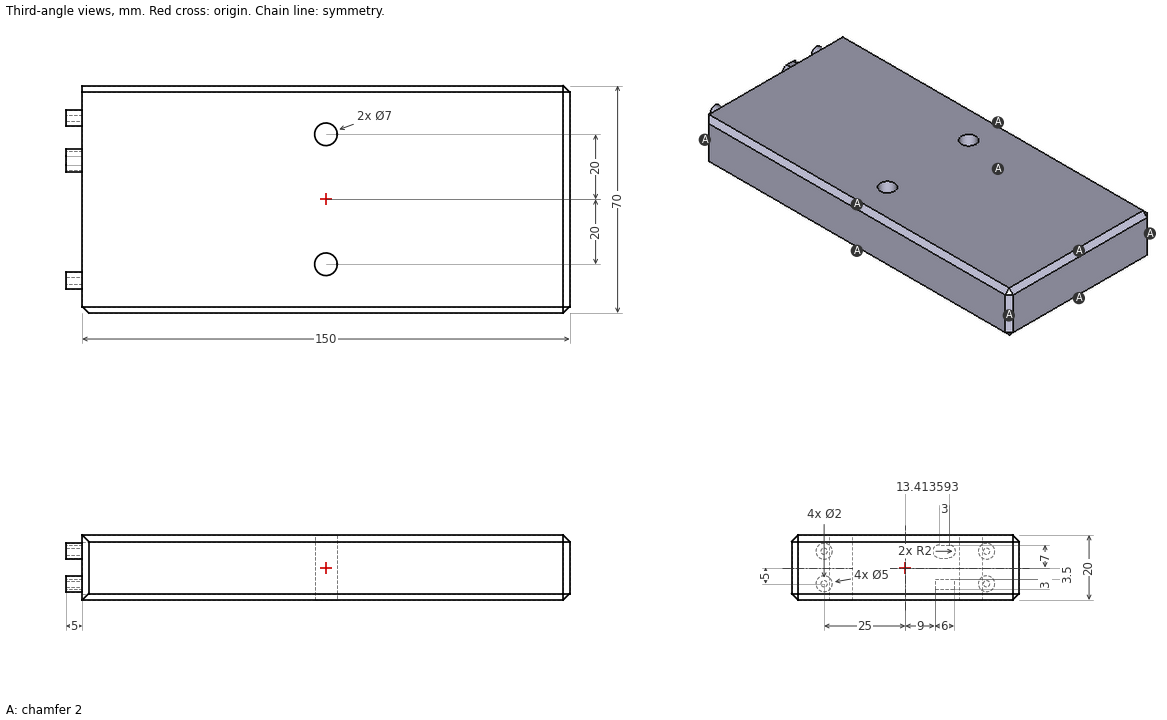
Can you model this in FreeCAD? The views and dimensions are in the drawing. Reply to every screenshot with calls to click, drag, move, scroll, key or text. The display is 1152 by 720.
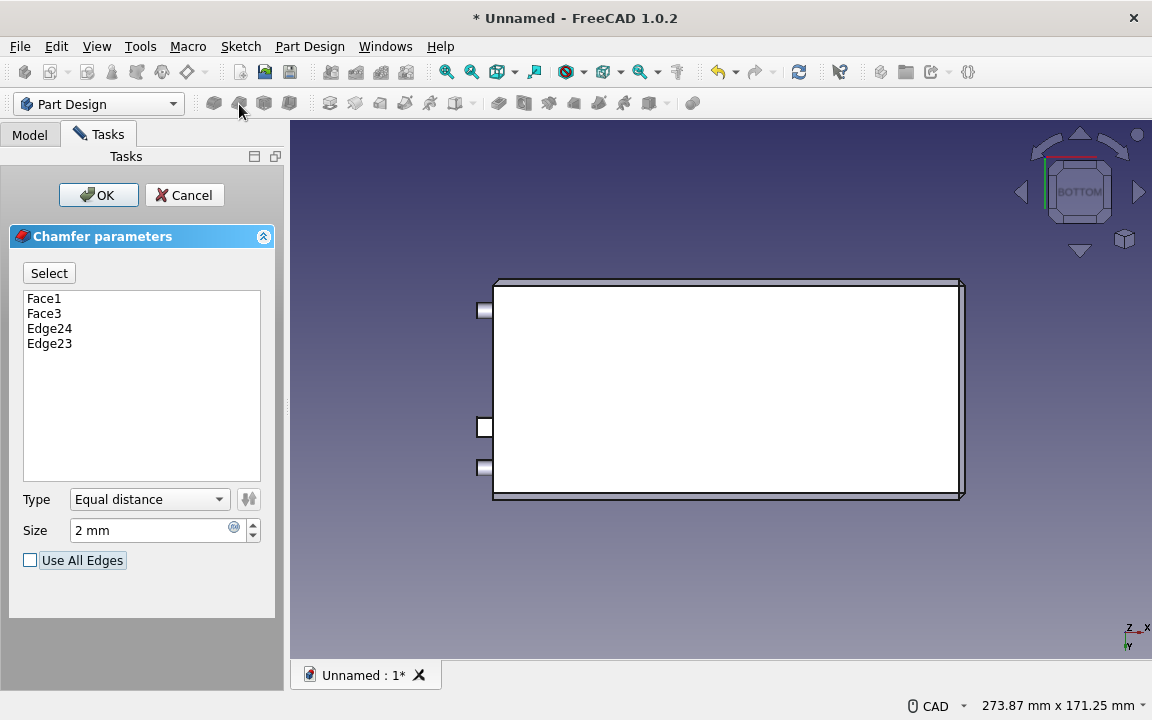
click(99, 195)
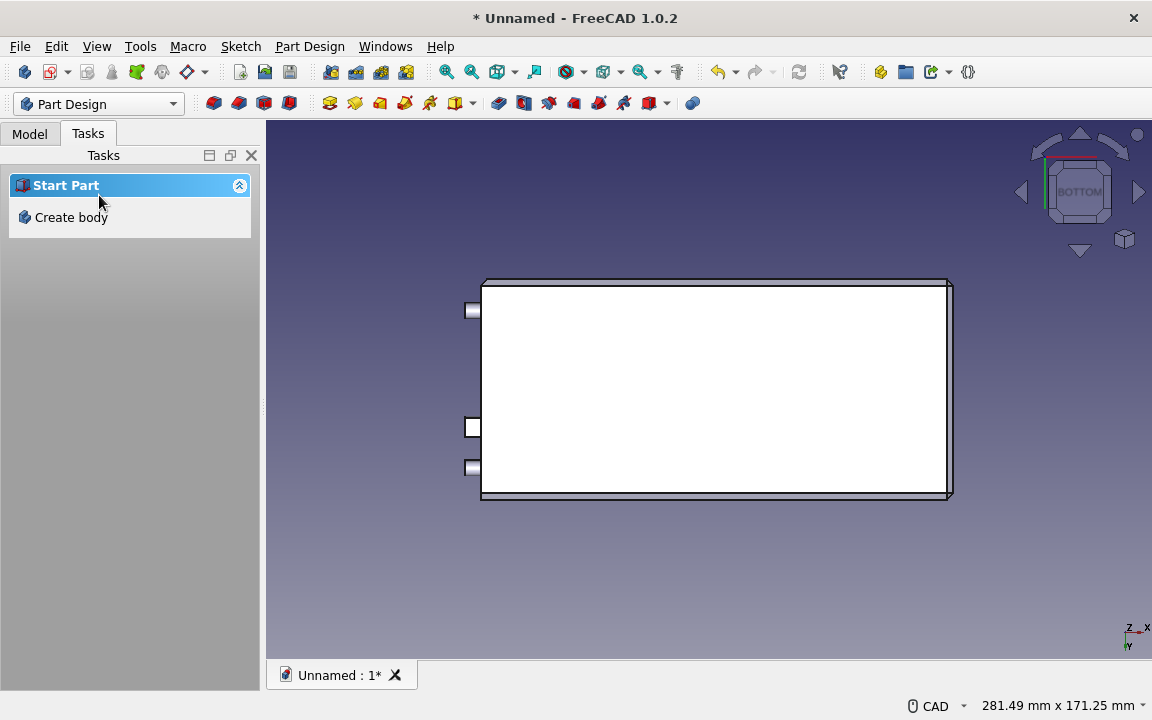
key(0)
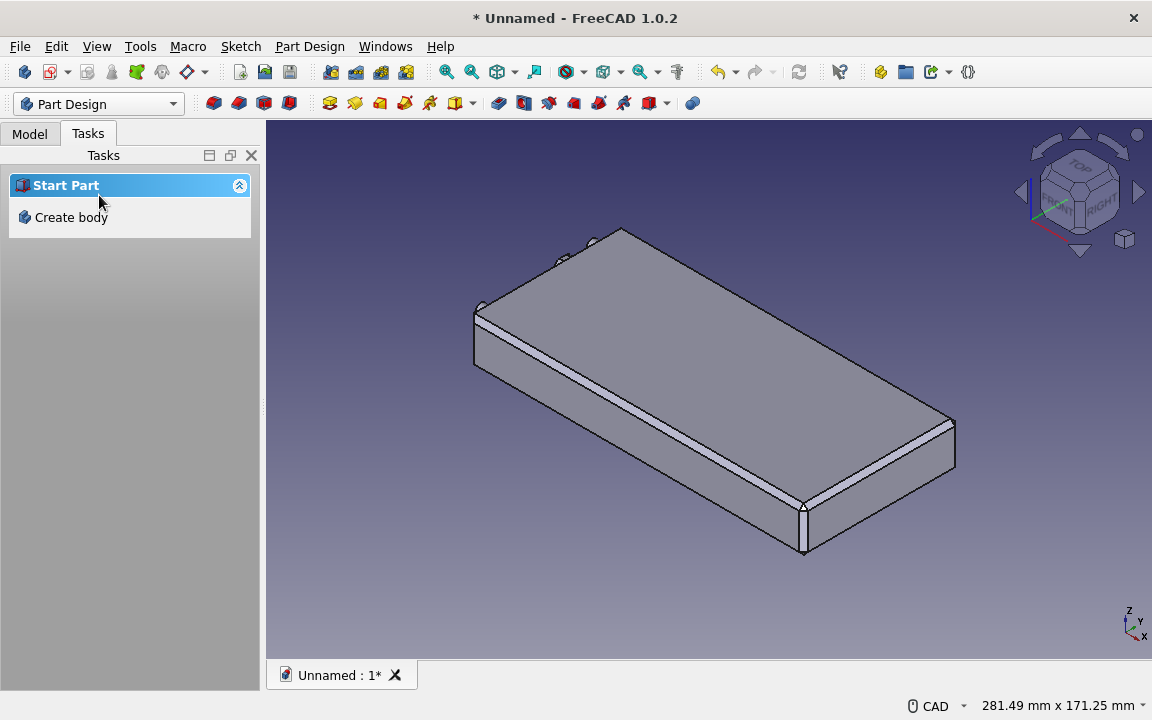
click(759, 392)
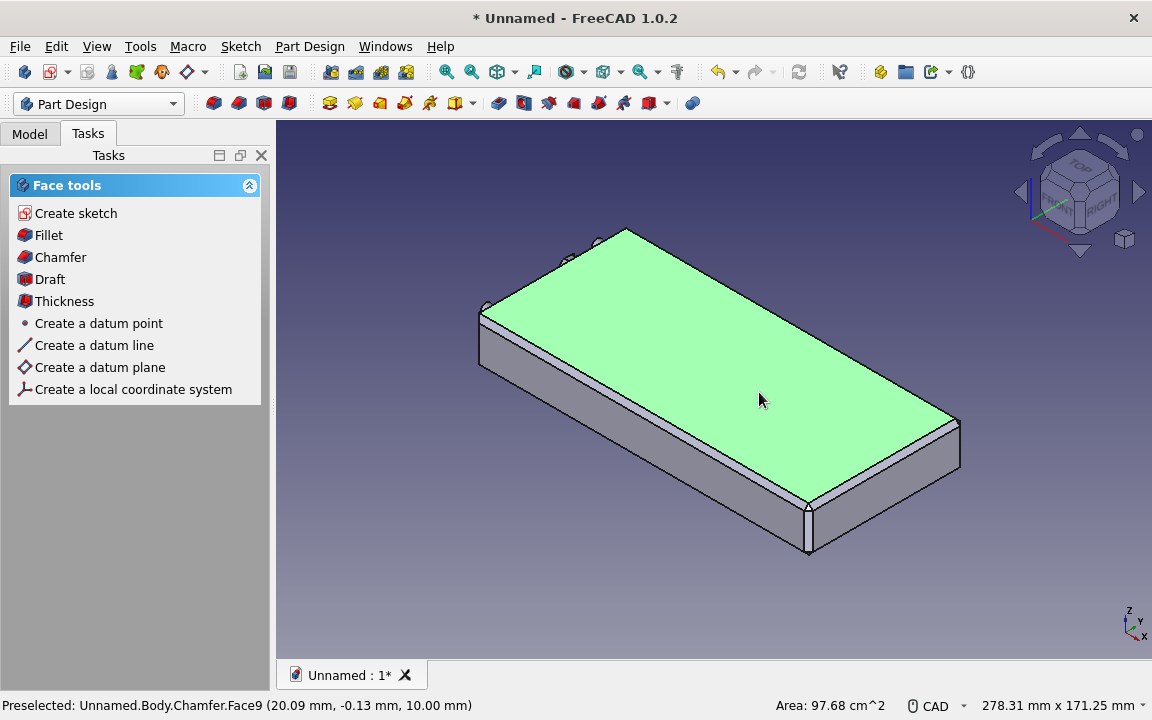
click(50, 72)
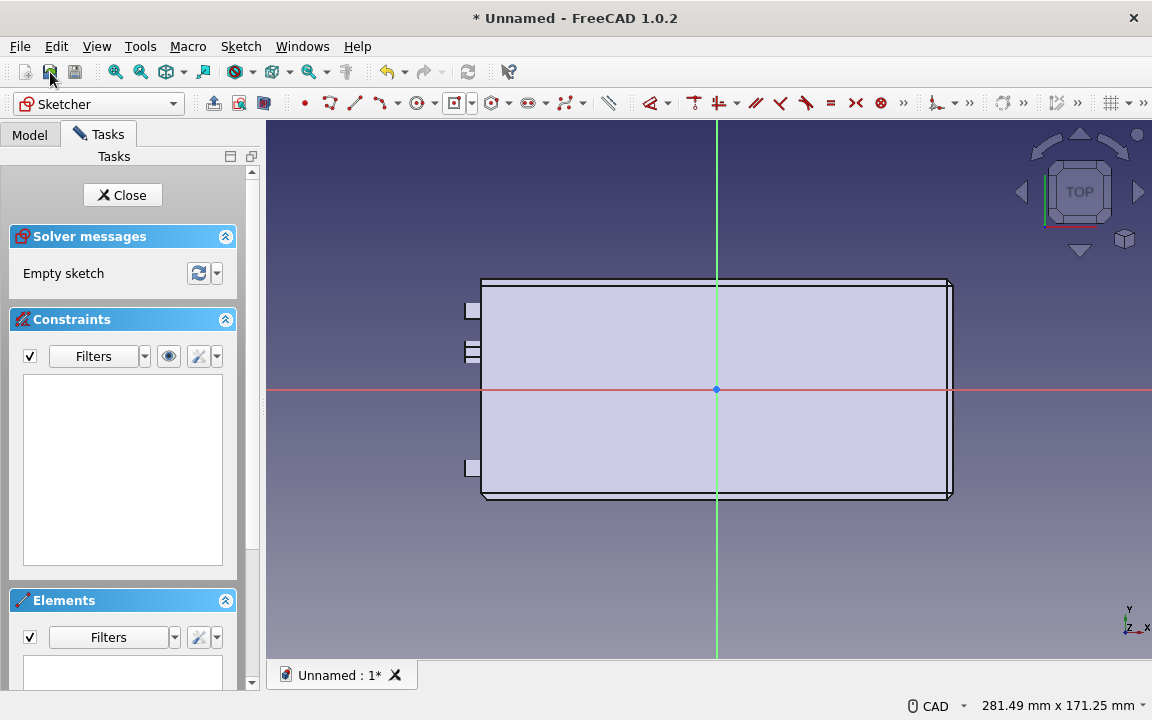
scroll(779, 390, up, 4)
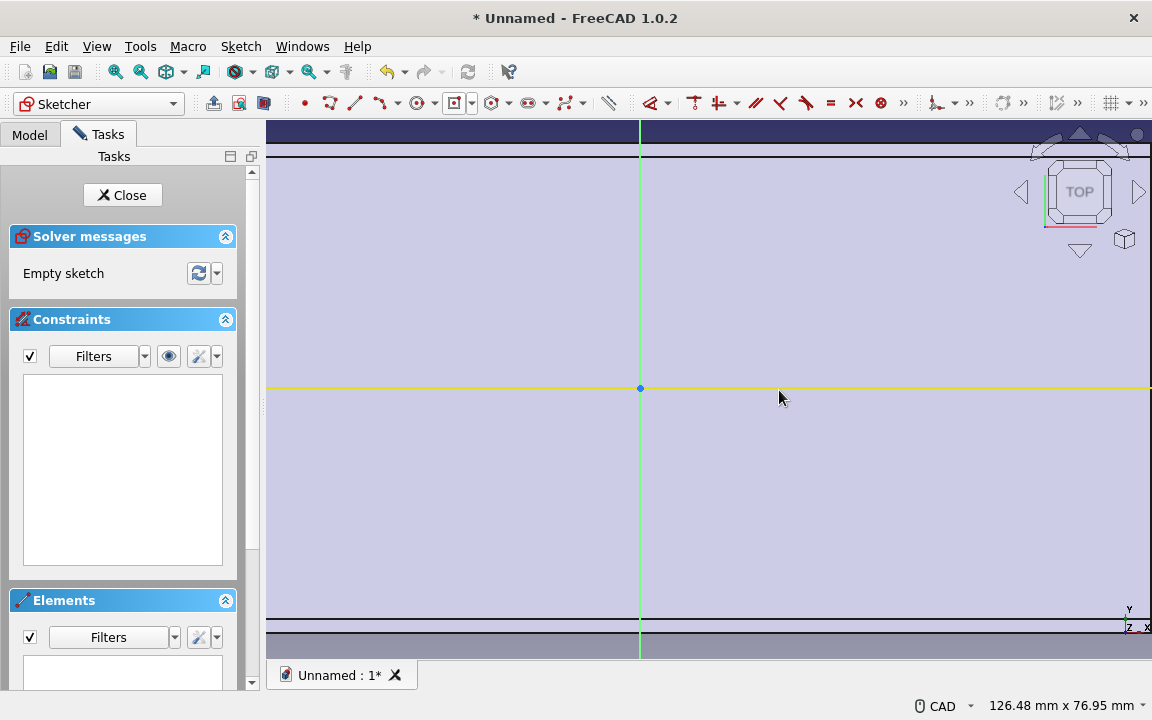
click(416, 104)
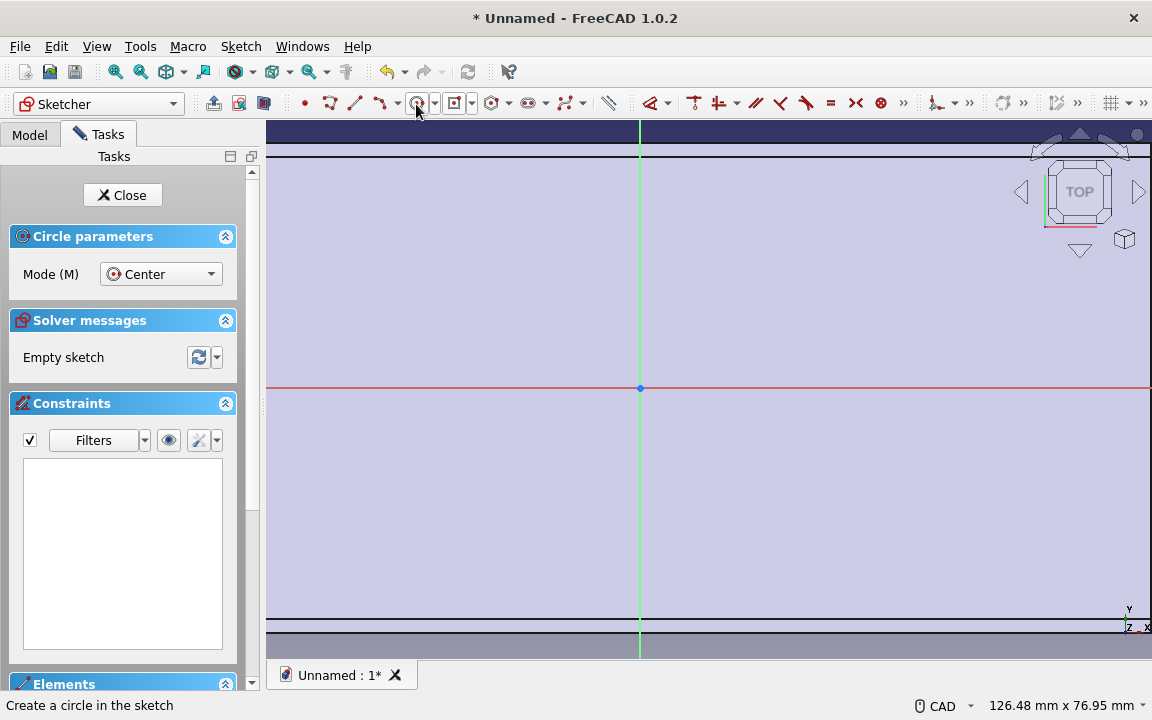
click(640, 248)
click(657, 231)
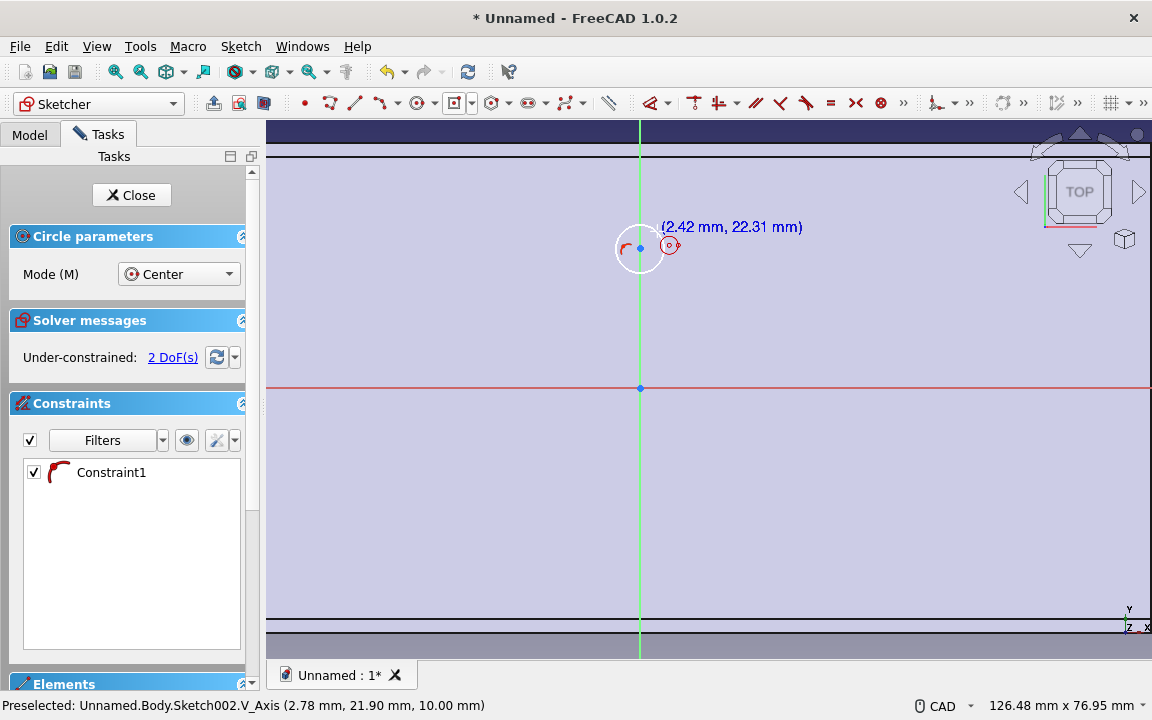
click(640, 528)
click(657, 511)
key(Escape)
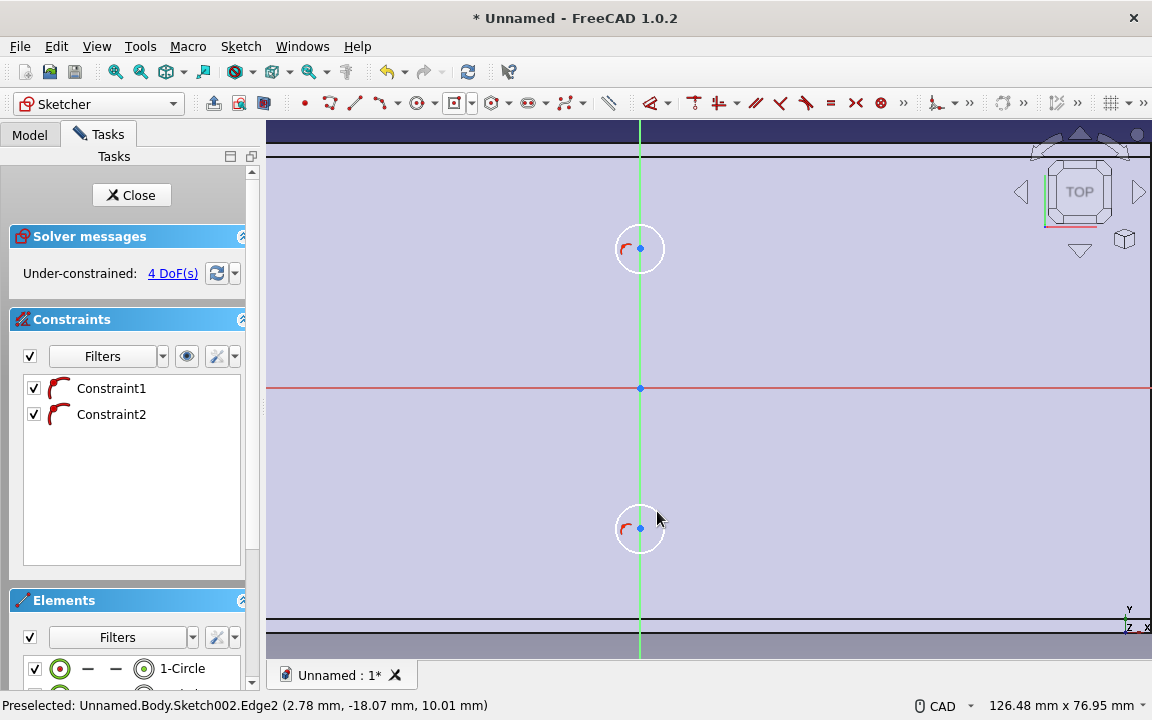
click(657, 232)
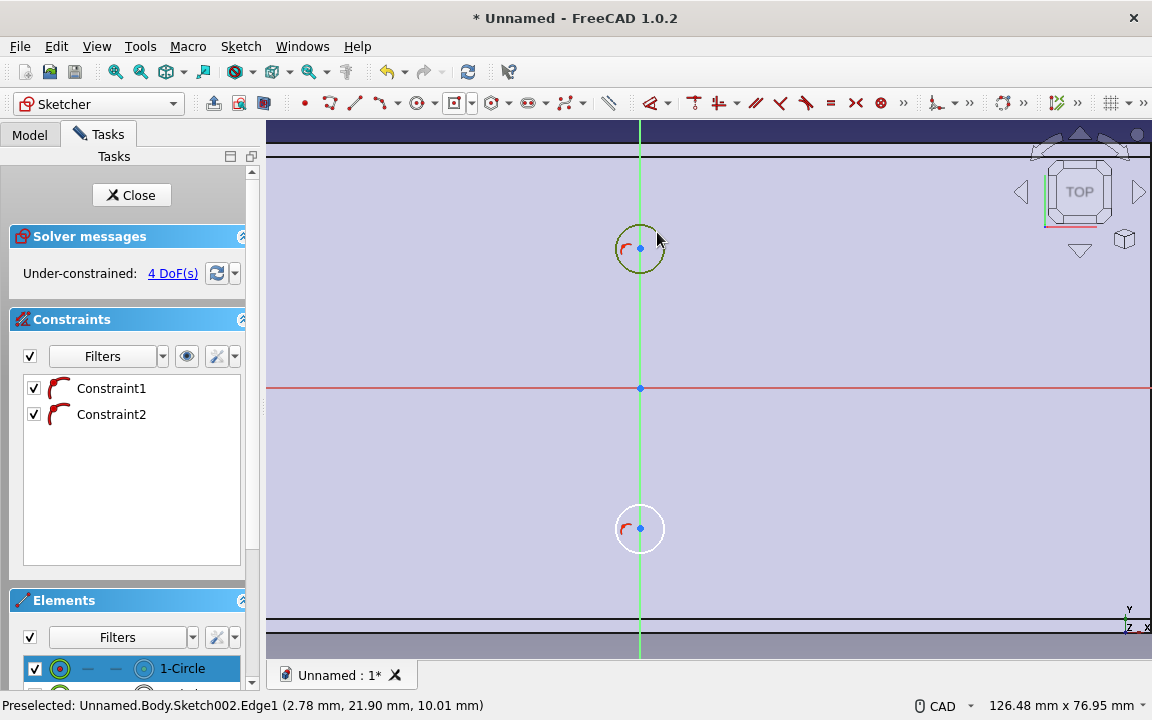
click(657, 512)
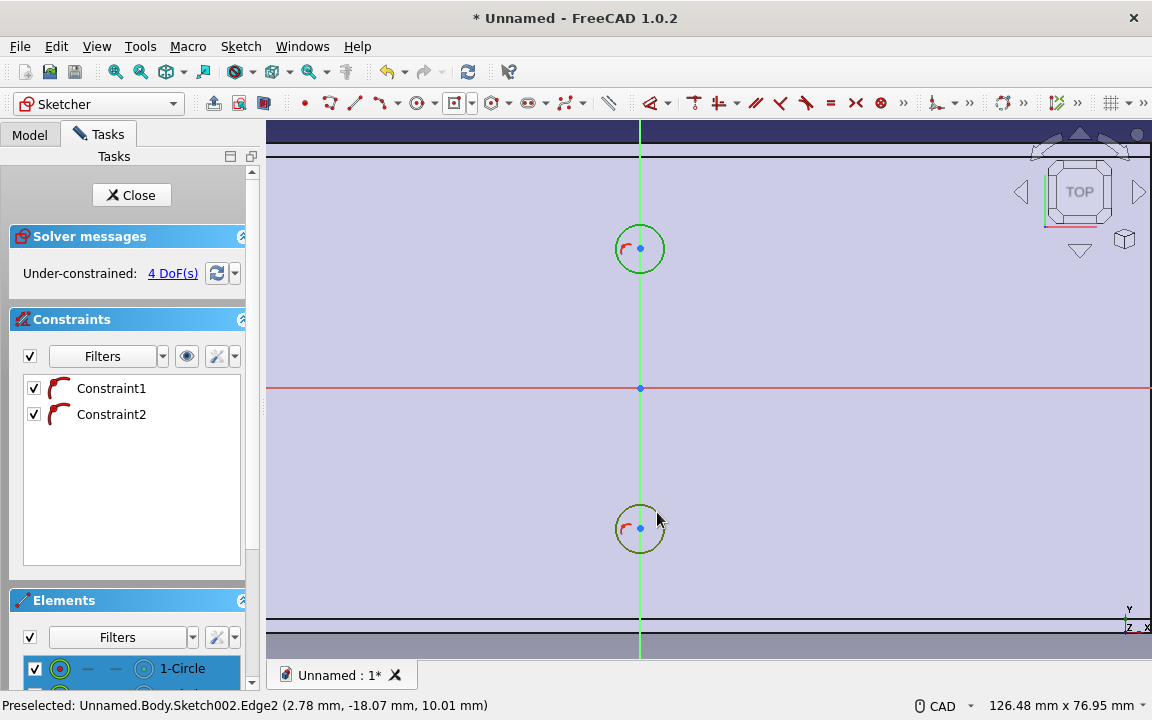
click(831, 104)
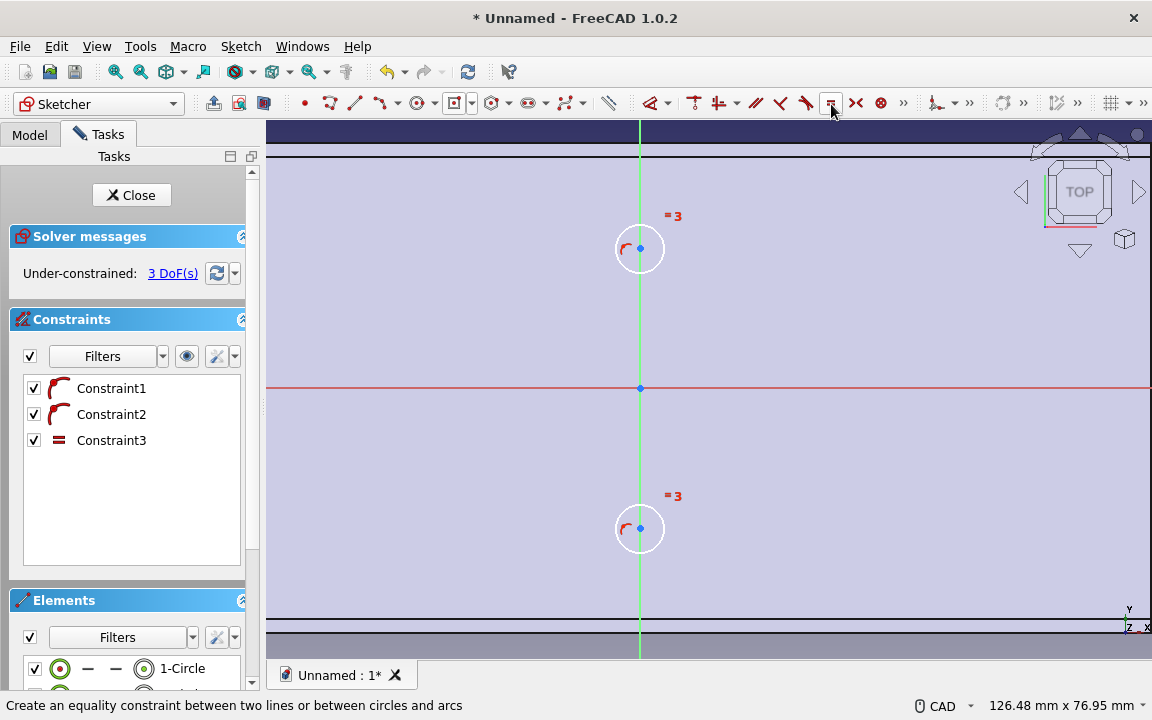
click(650, 104)